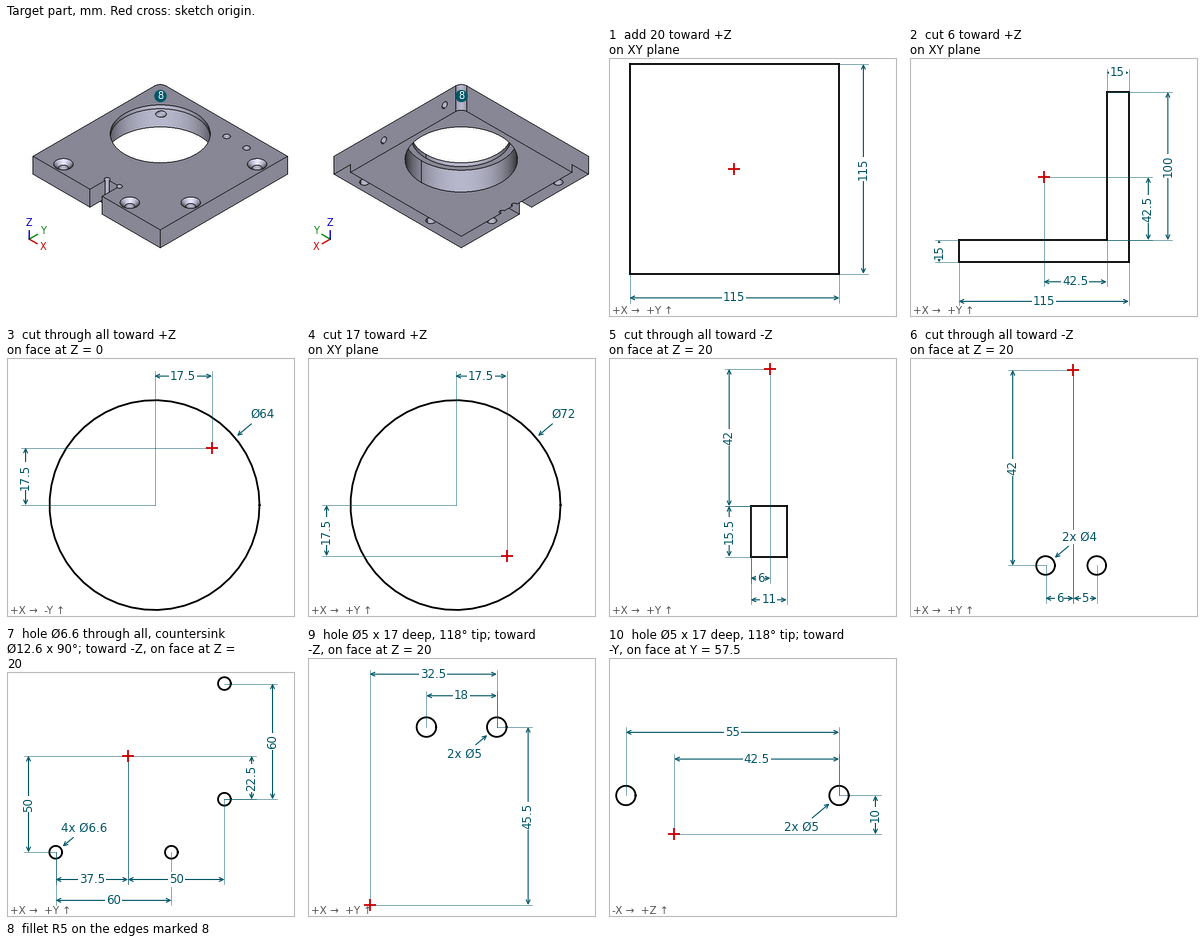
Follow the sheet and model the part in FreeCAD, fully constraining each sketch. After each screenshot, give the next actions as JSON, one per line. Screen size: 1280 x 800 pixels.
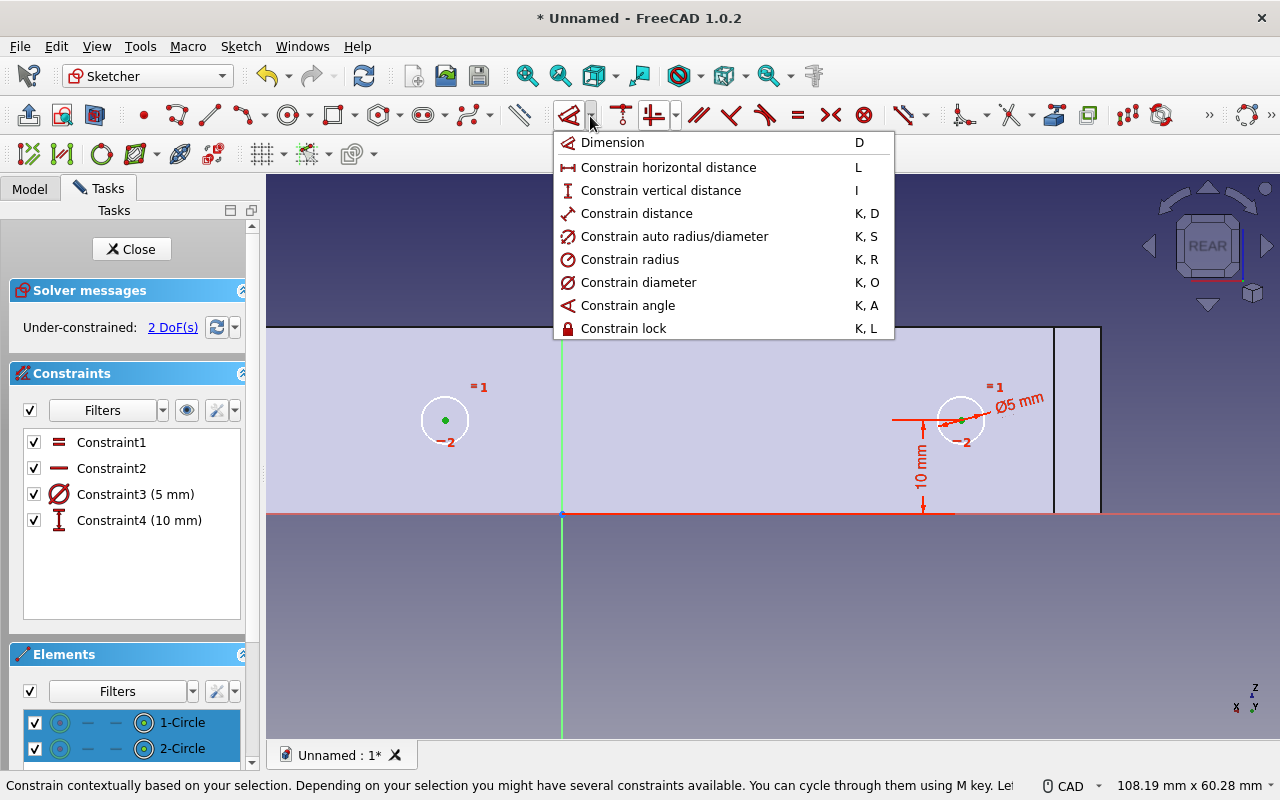
{"action": "left_click", "coordinate": [724, 168]}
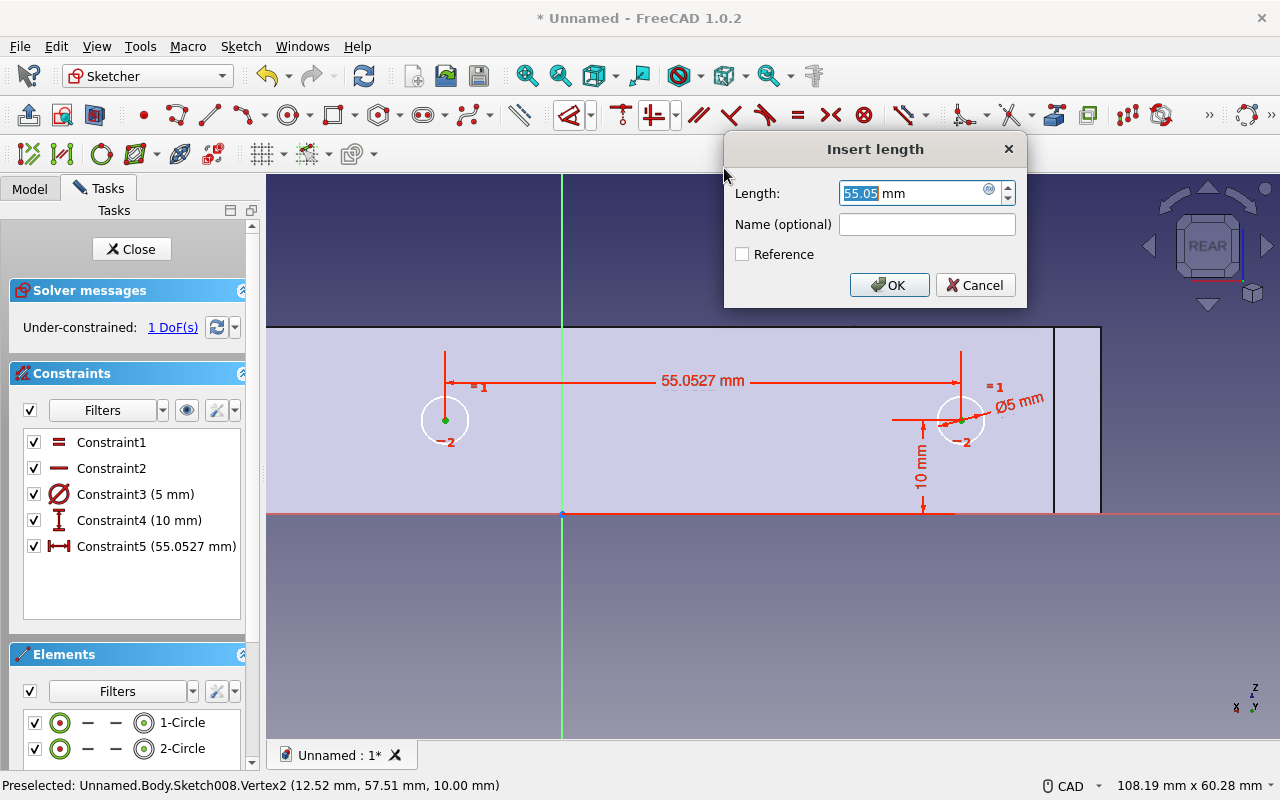
{"action": "type", "text": "55"}
{"action": "key", "text": "Return"}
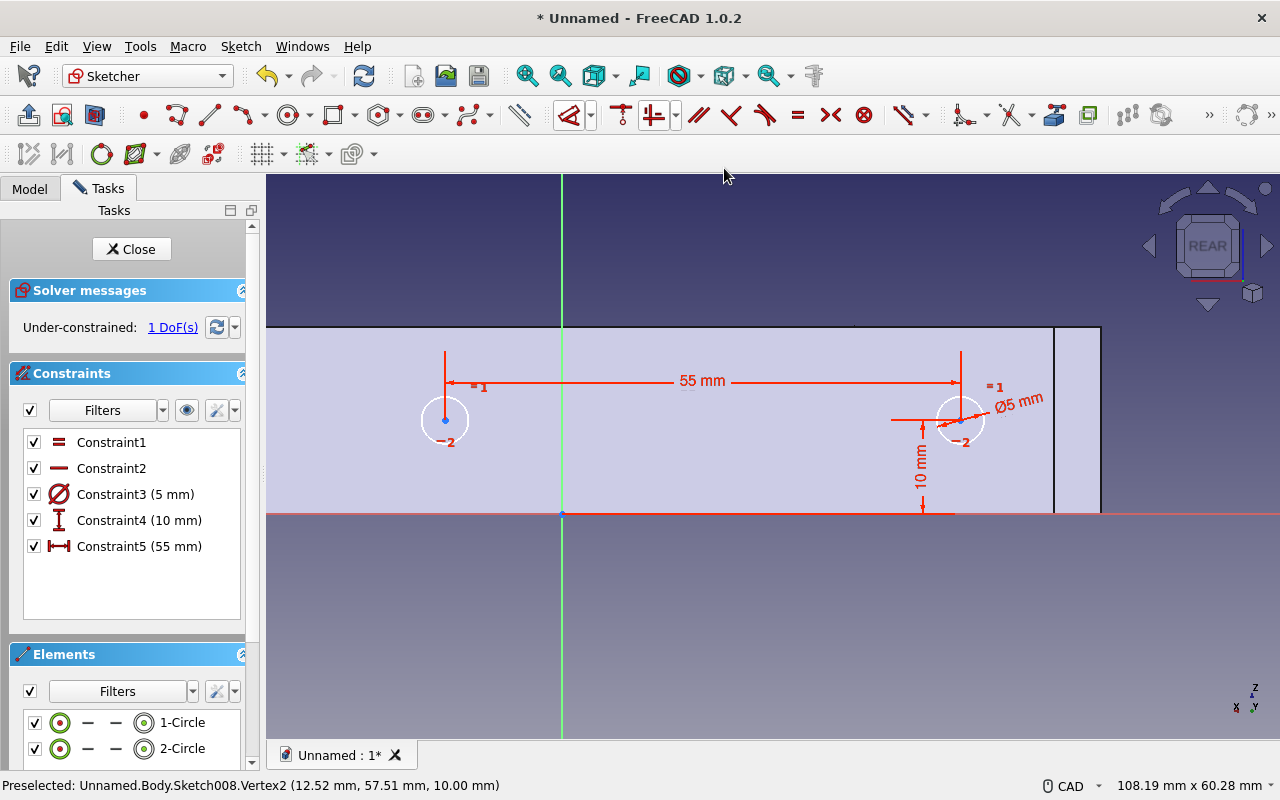
{"action": "left_click", "coordinate": [961, 420]}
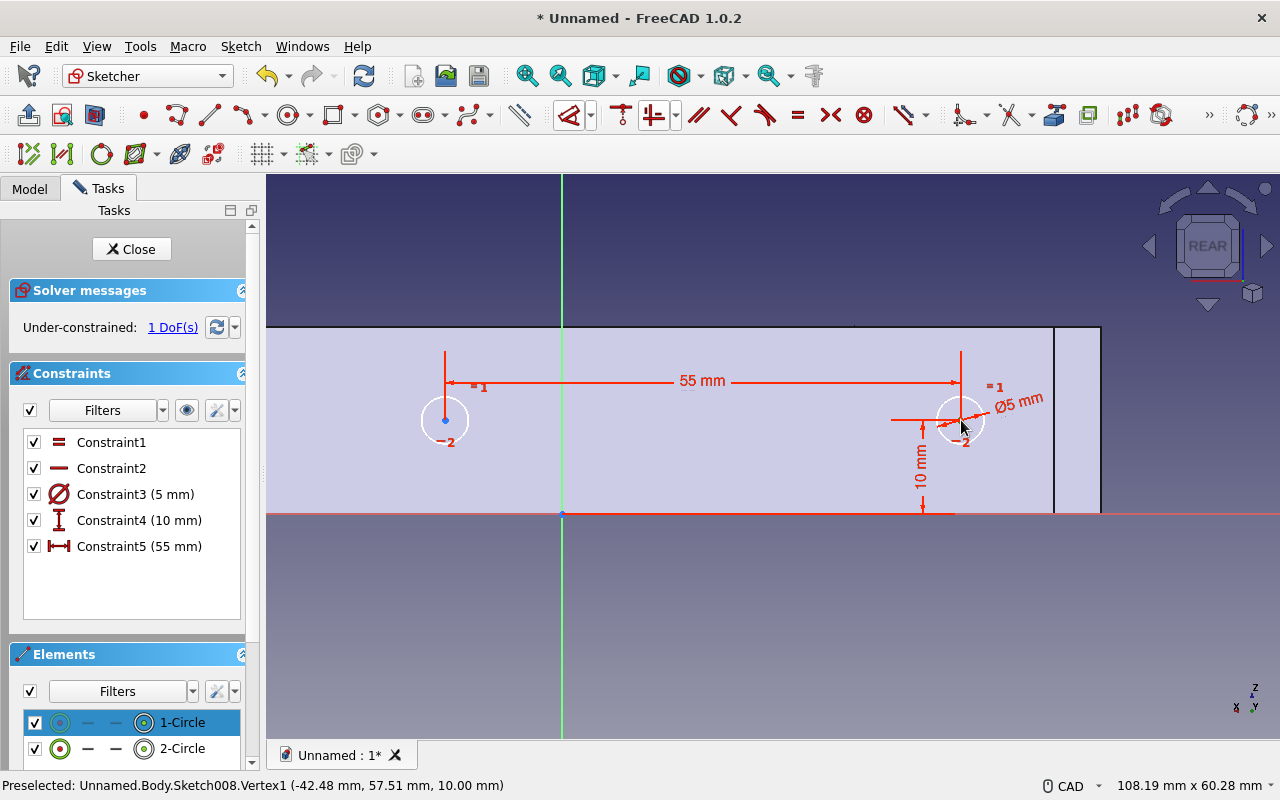
{"action": "key", "text": "l"}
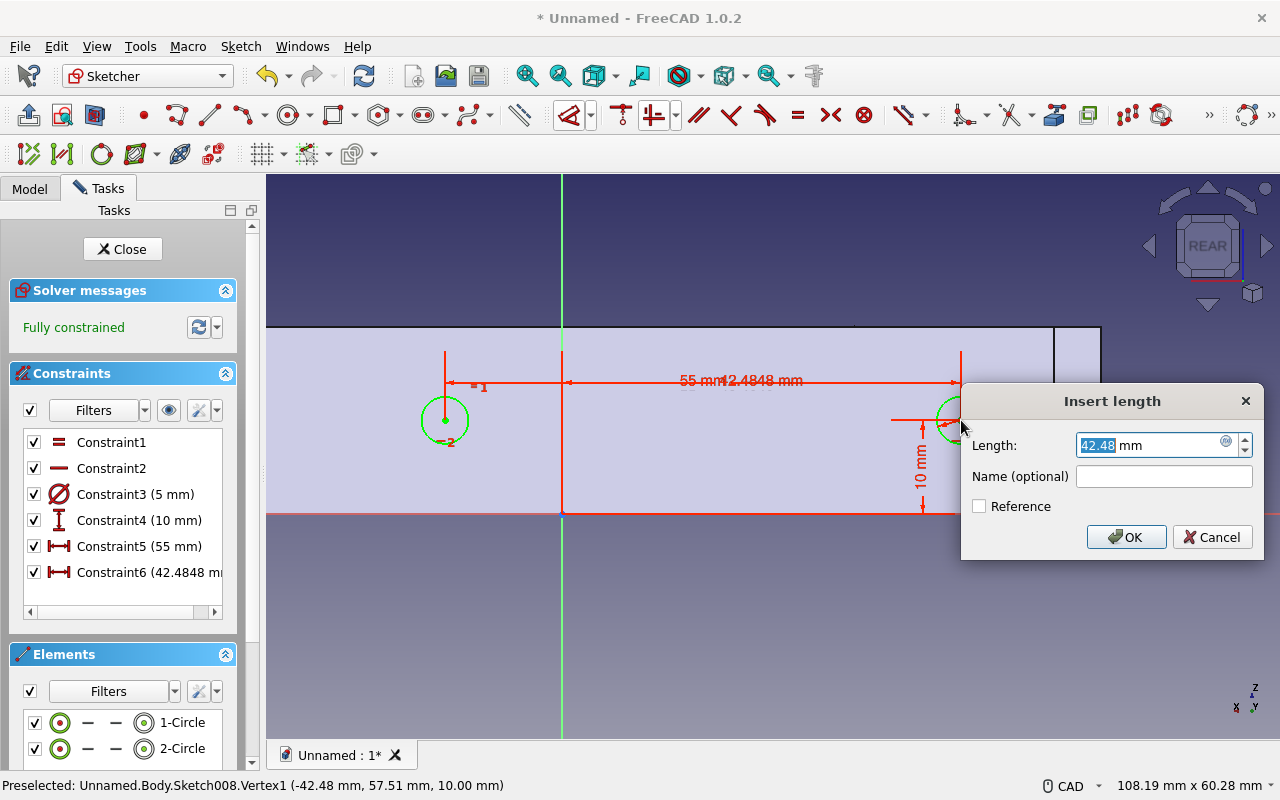
{"action": "type", "text": "42.5"}
{"action": "key", "text": "Return"}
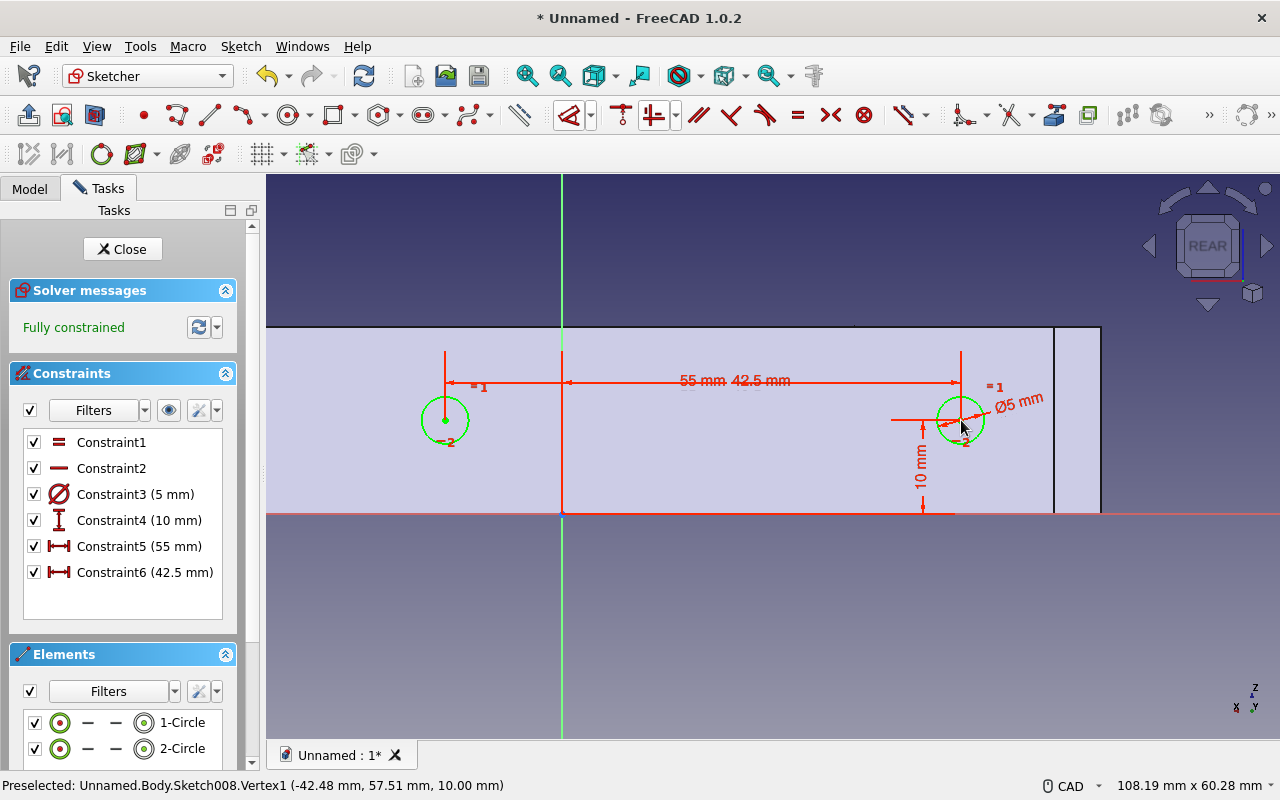
{"action": "left_click", "coordinate": [123, 249]}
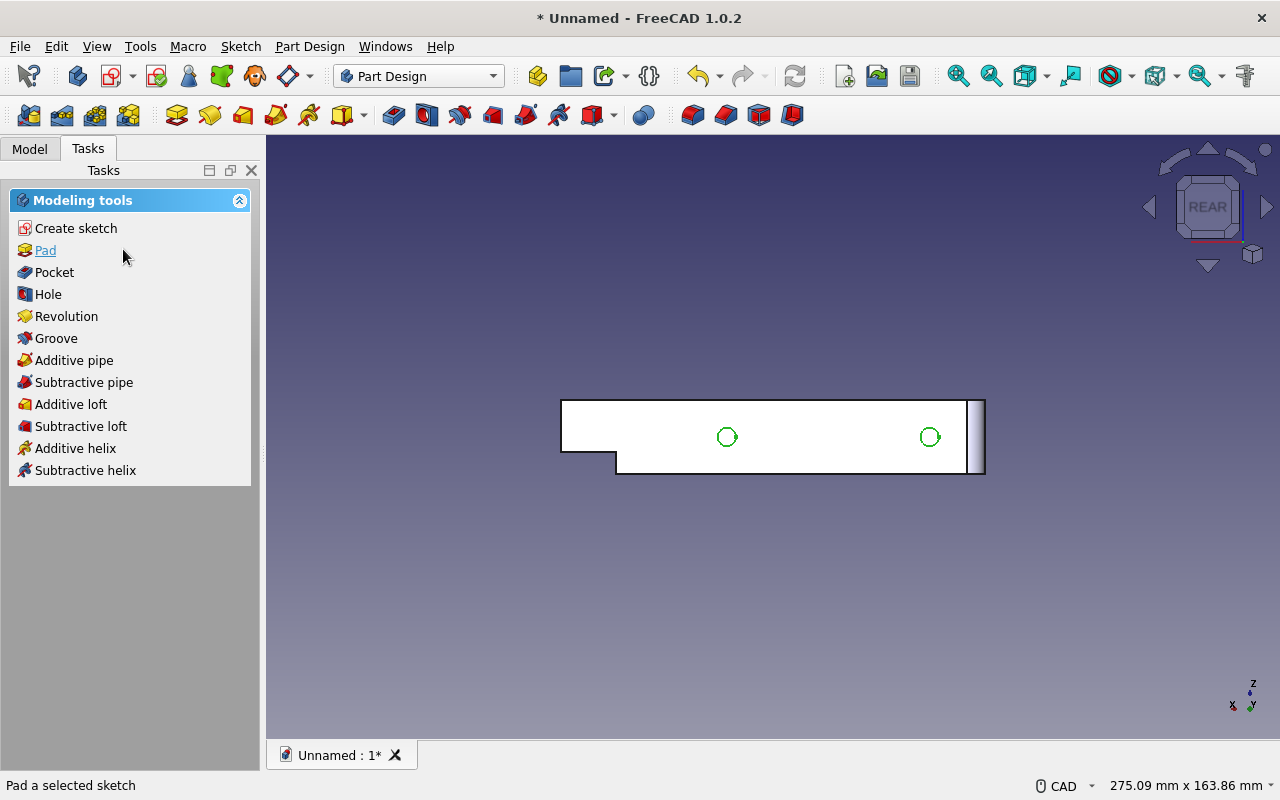
{"action": "left_click", "coordinate": [427, 116]}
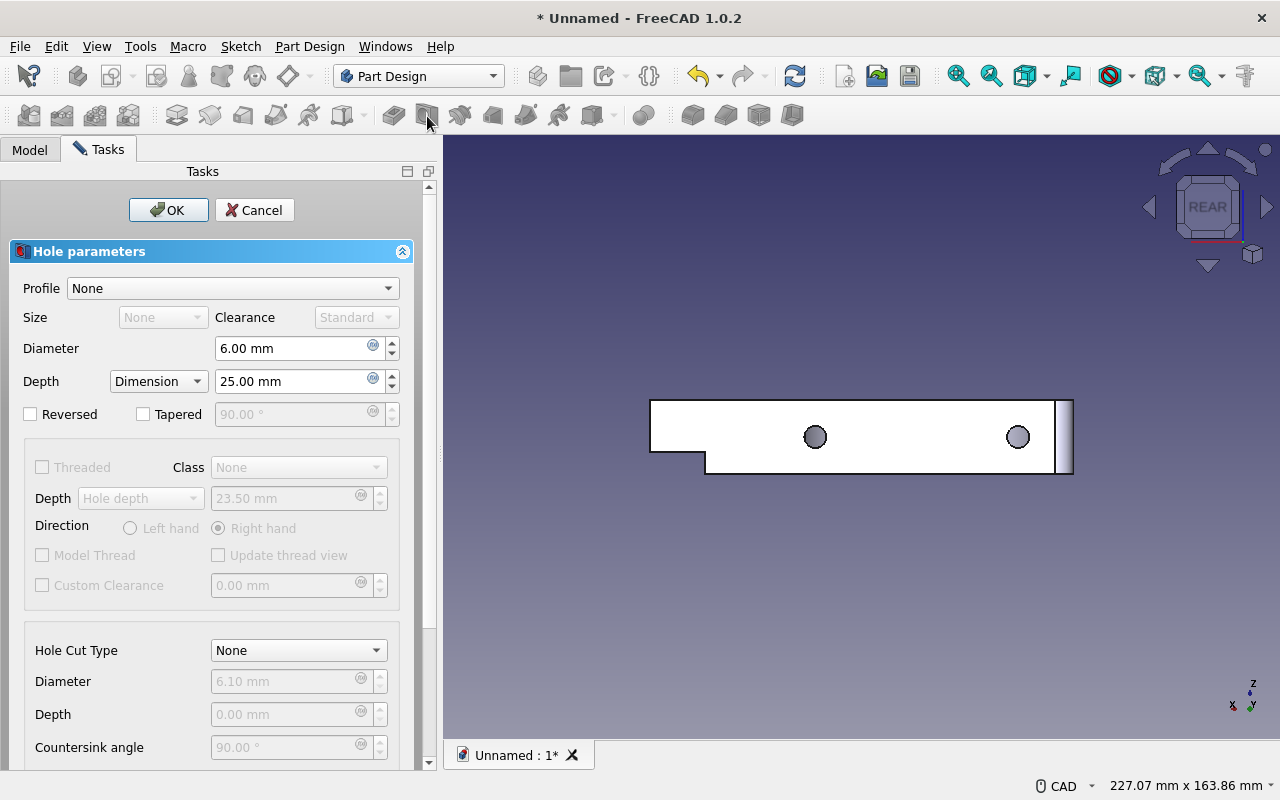
{"action": "triple_click", "coordinate": [300, 348]}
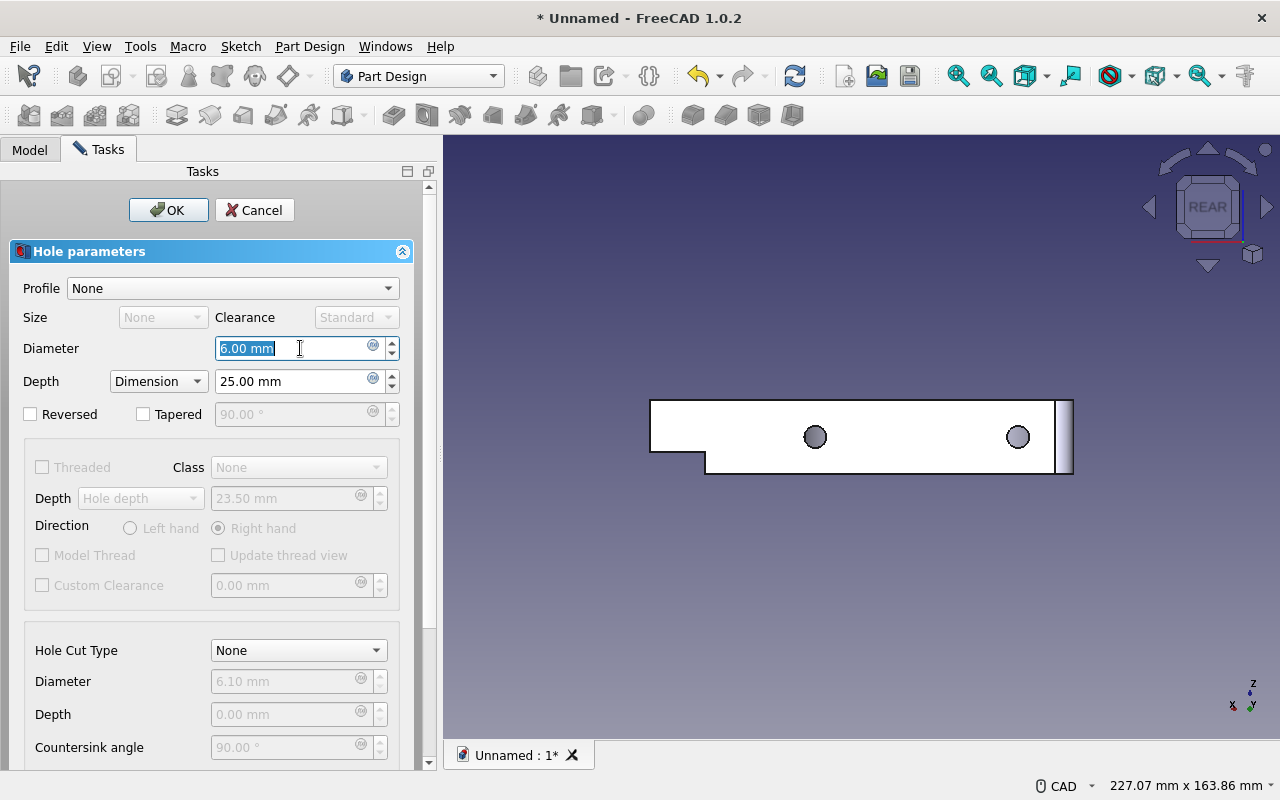
{"action": "type", "text": "5"}
{"action": "key", "text": "Tab"}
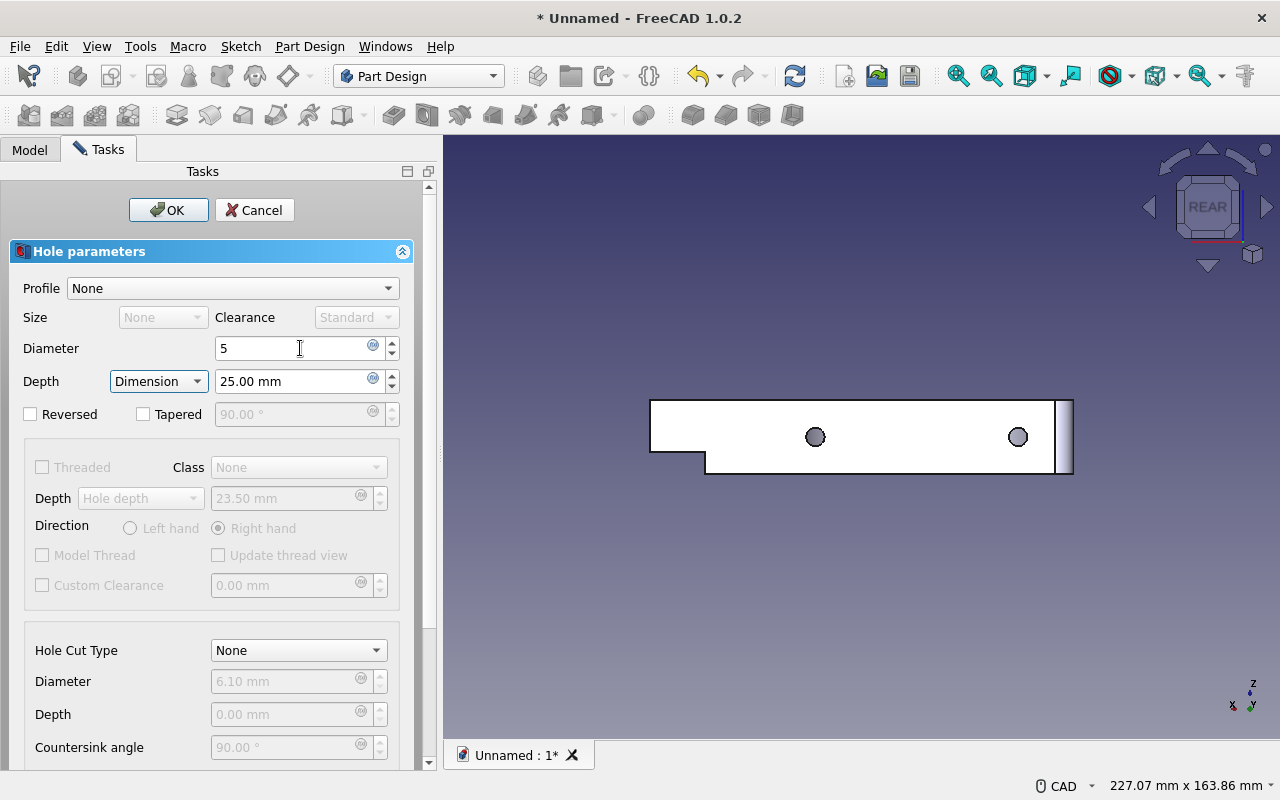
{"action": "triple_click", "coordinate": [300, 382]}